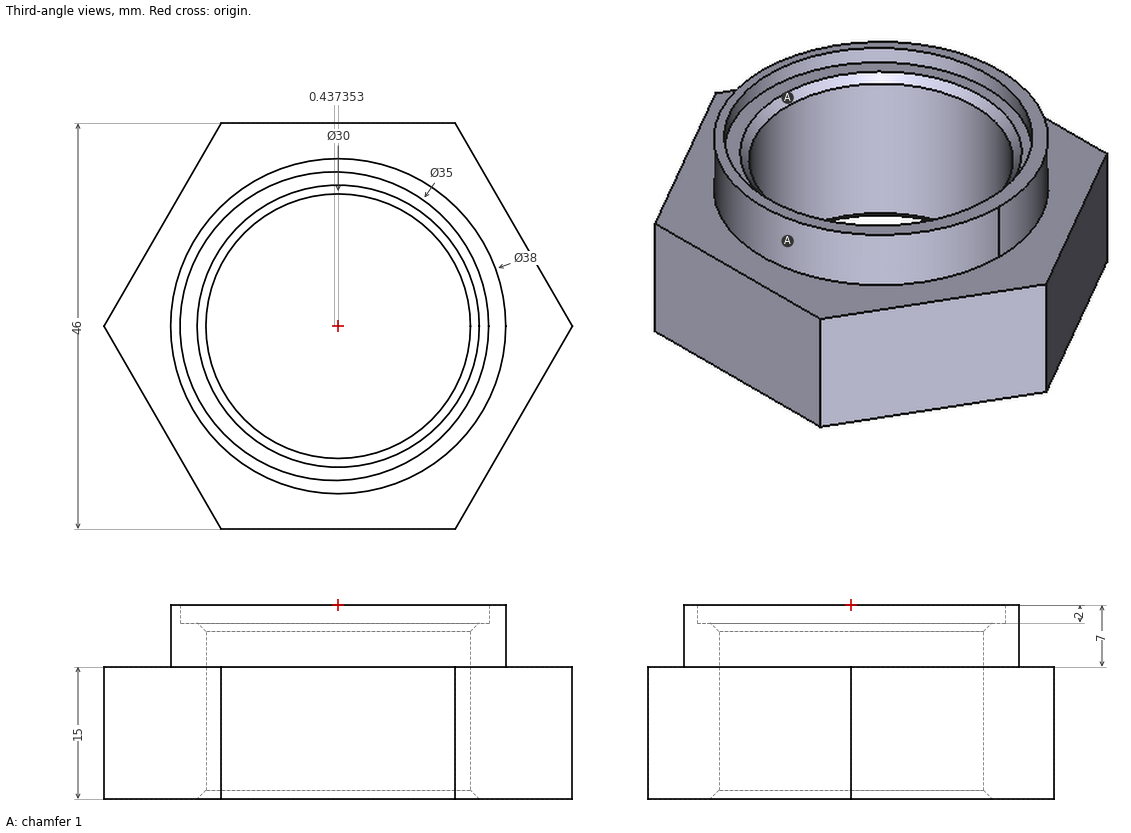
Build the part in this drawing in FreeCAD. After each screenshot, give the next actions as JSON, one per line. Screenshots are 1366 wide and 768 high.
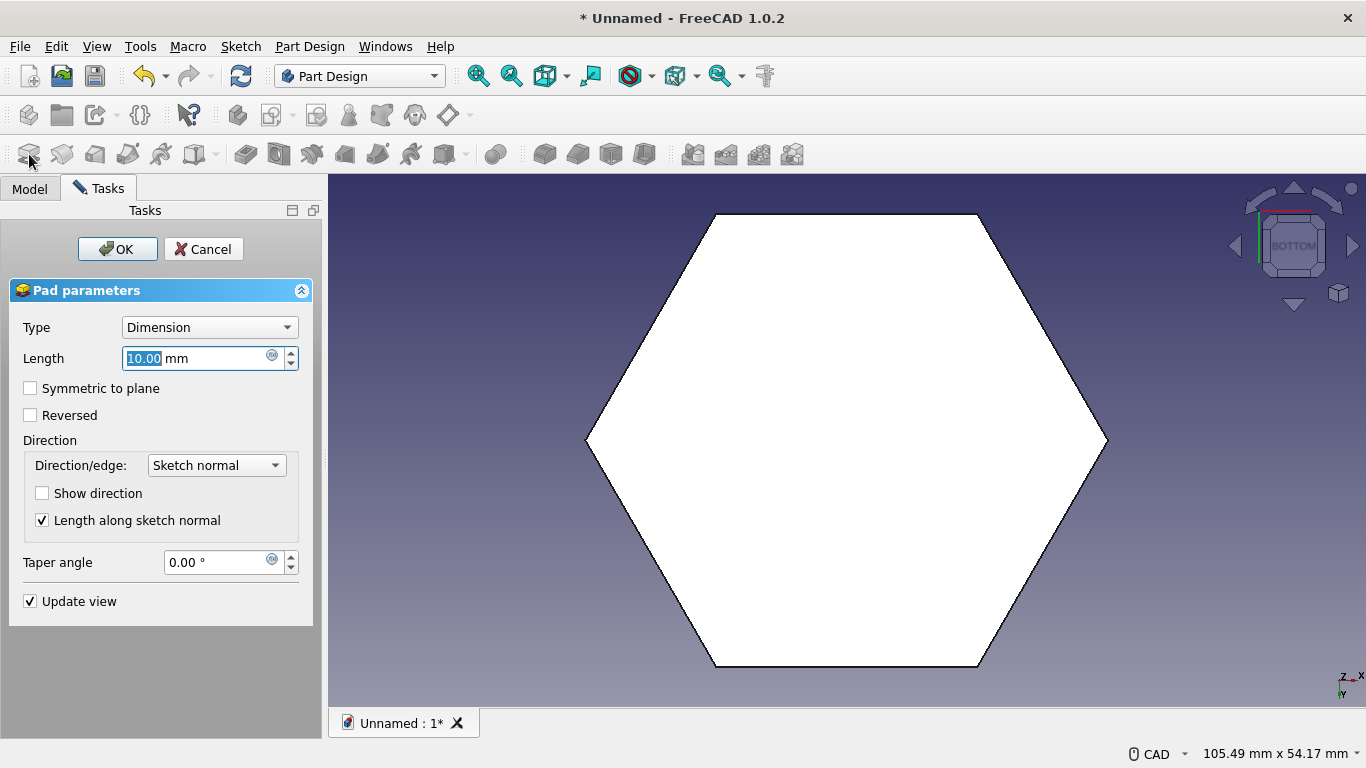
{"action": "type", "text": "15"}
{"action": "key", "text": "Tab"}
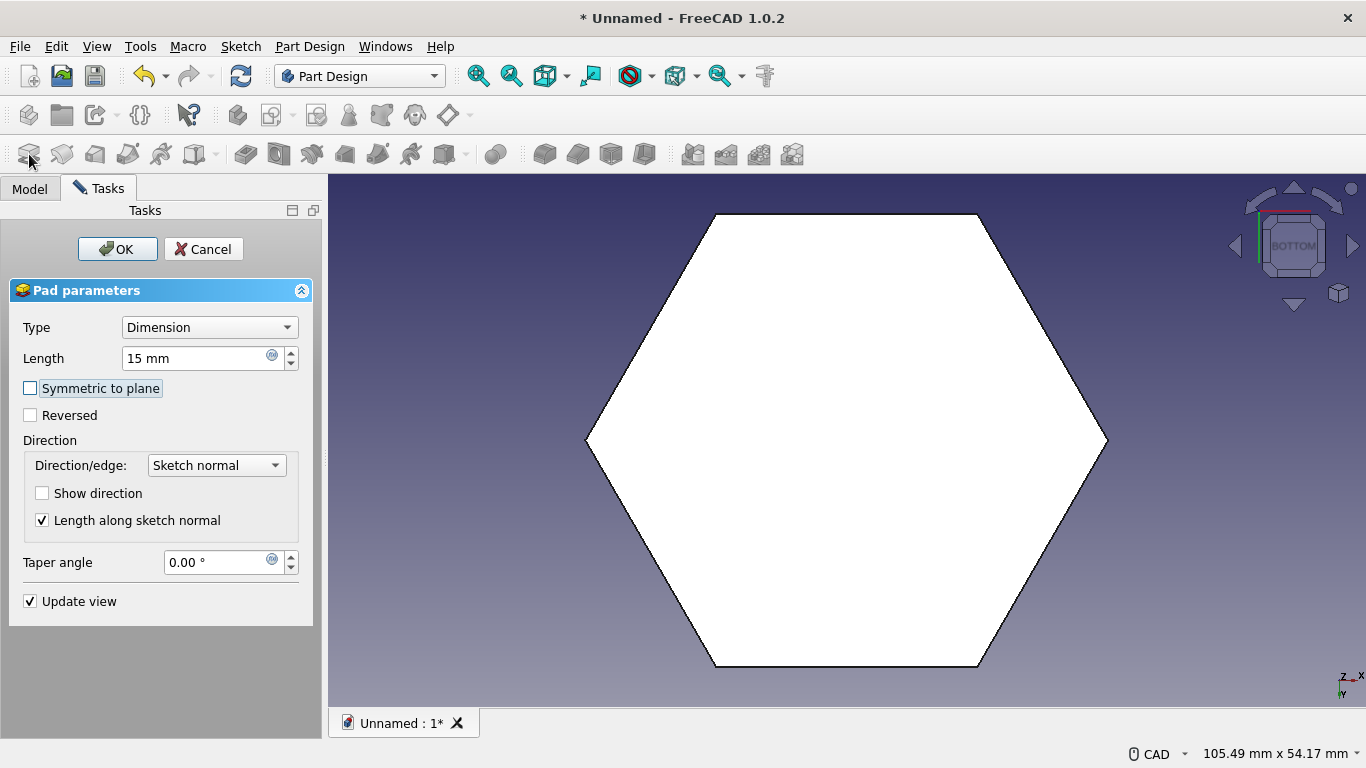
{"action": "left_click", "coordinate": [118, 249]}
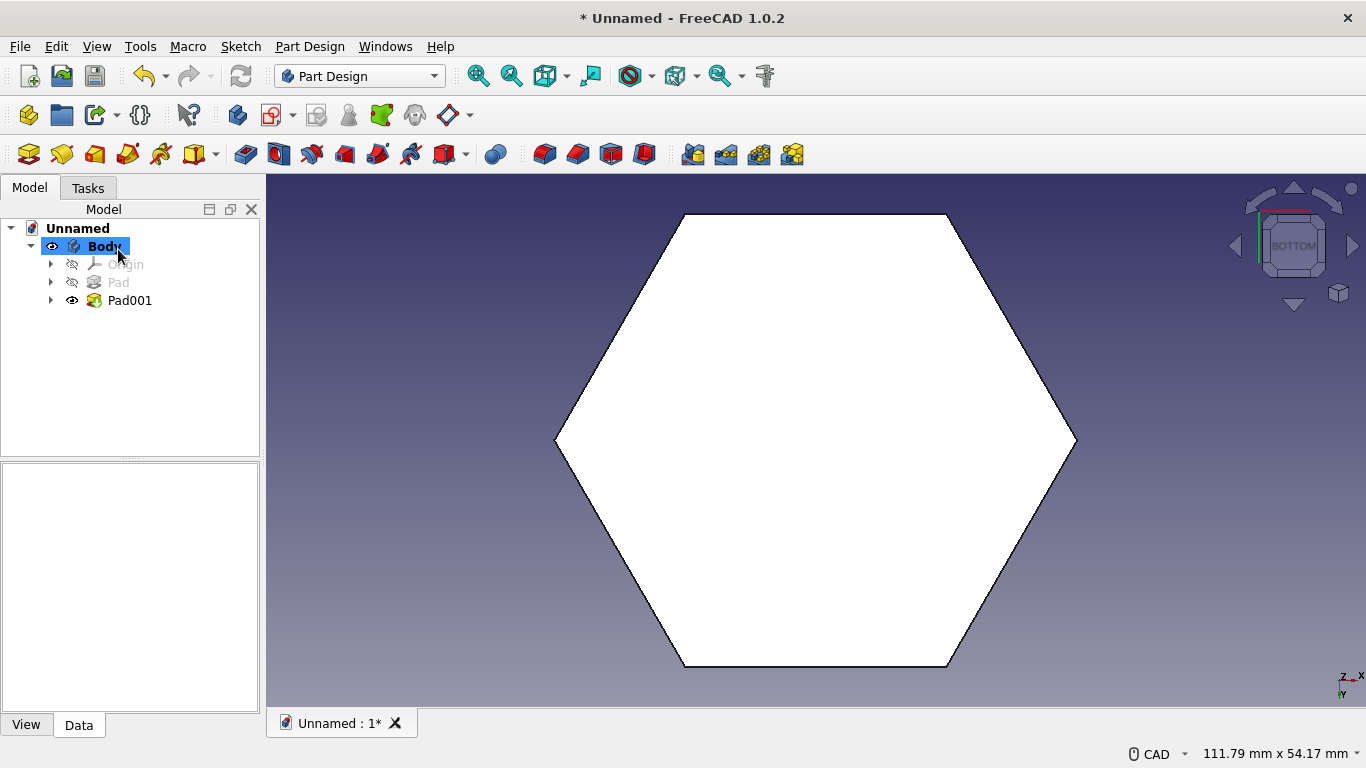
{"action": "left_click", "coordinate": [270, 116]}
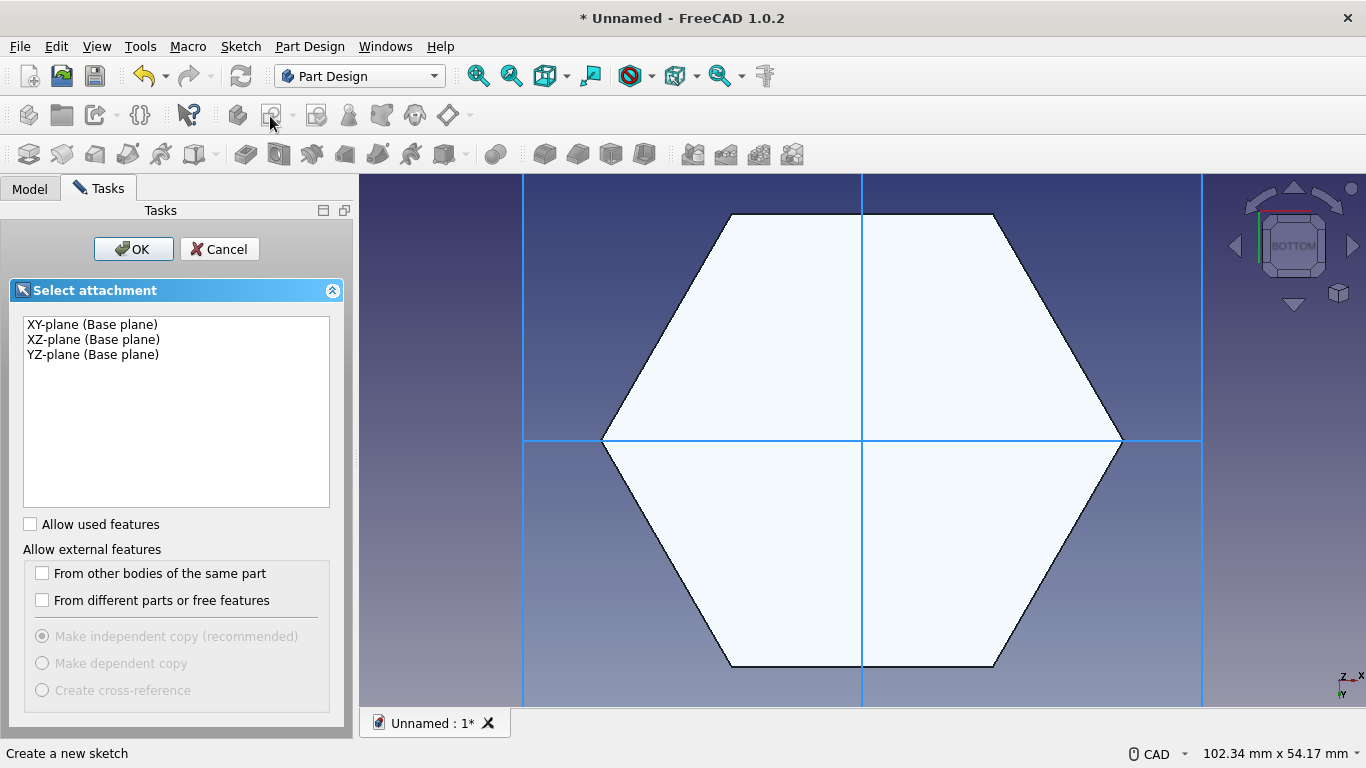
{"action": "left_click", "coordinate": [84, 324]}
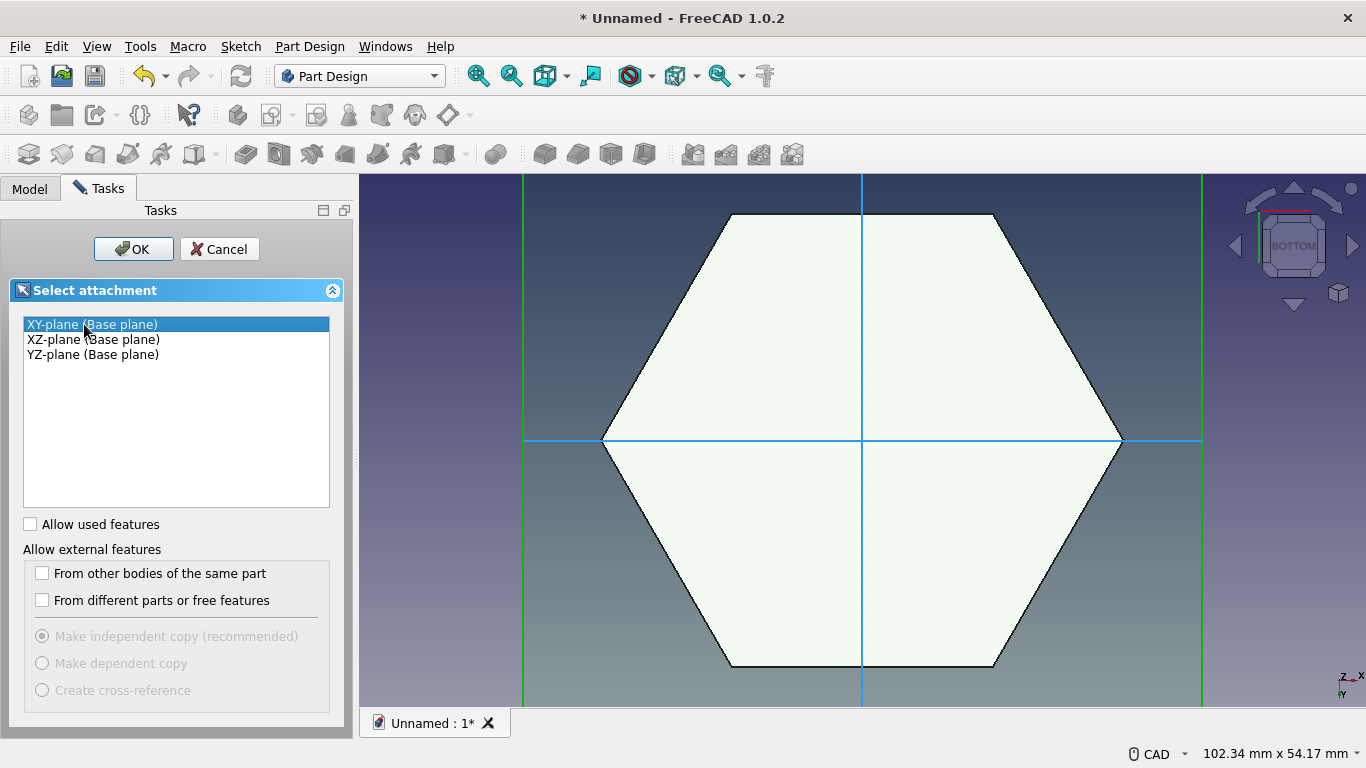
{"action": "left_click", "coordinate": [134, 249]}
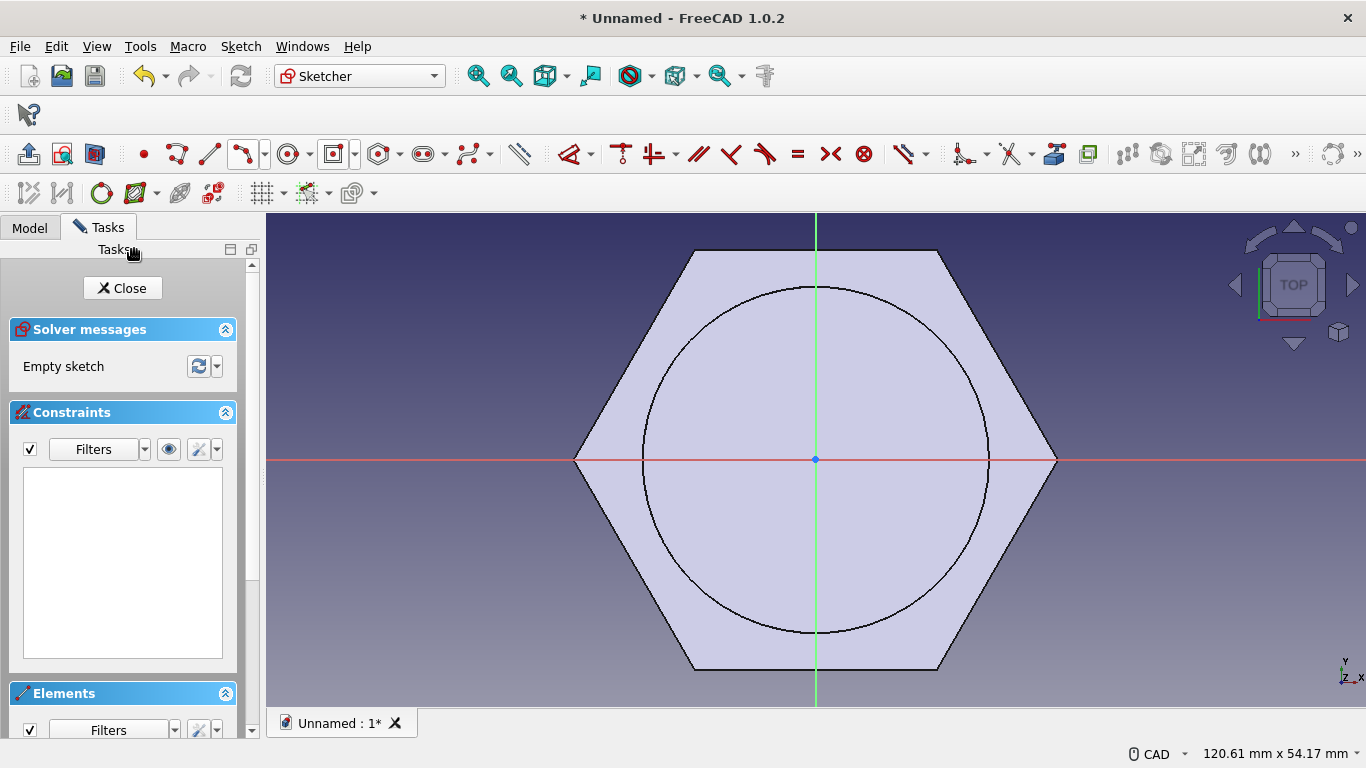
{"action": "left_click", "coordinate": [288, 154]}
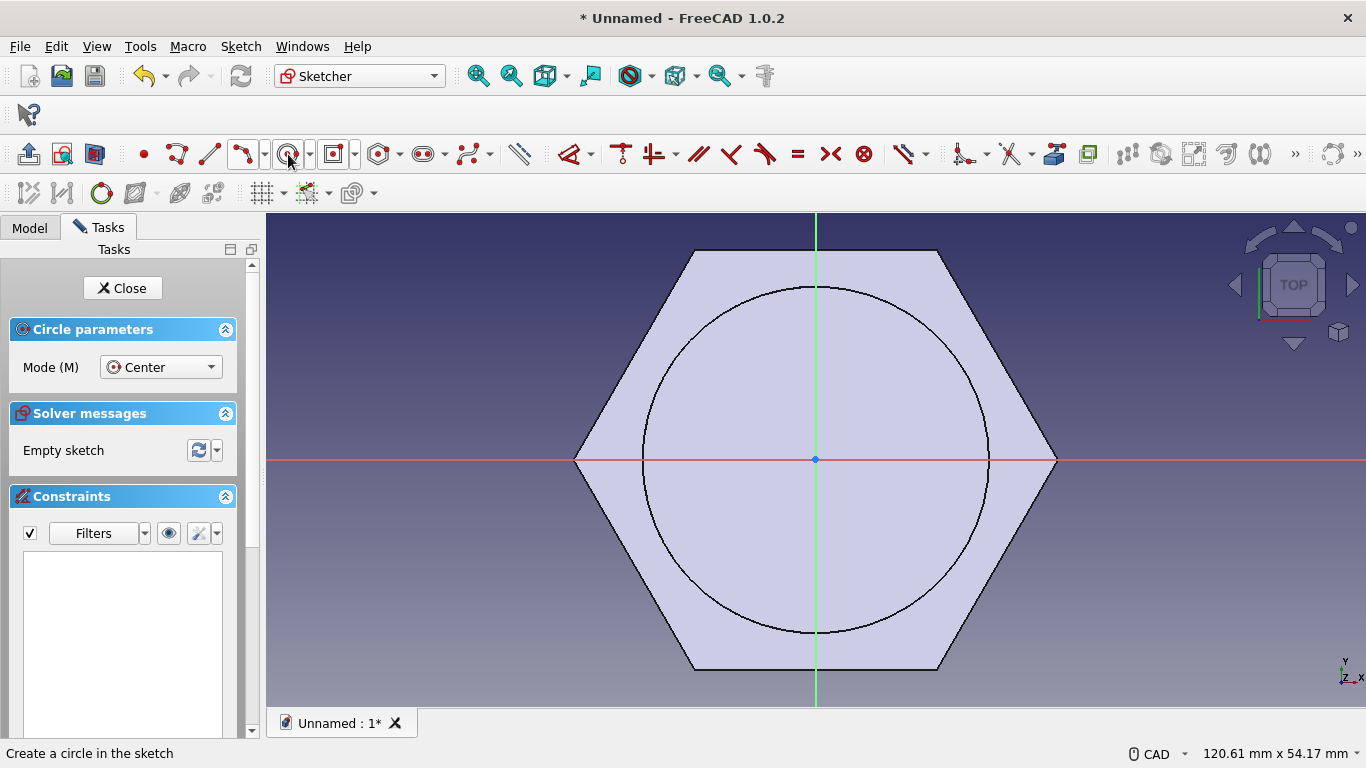
{"action": "scroll", "coordinate": [812, 460], "scroll_direction": "up", "scroll_amount": 7}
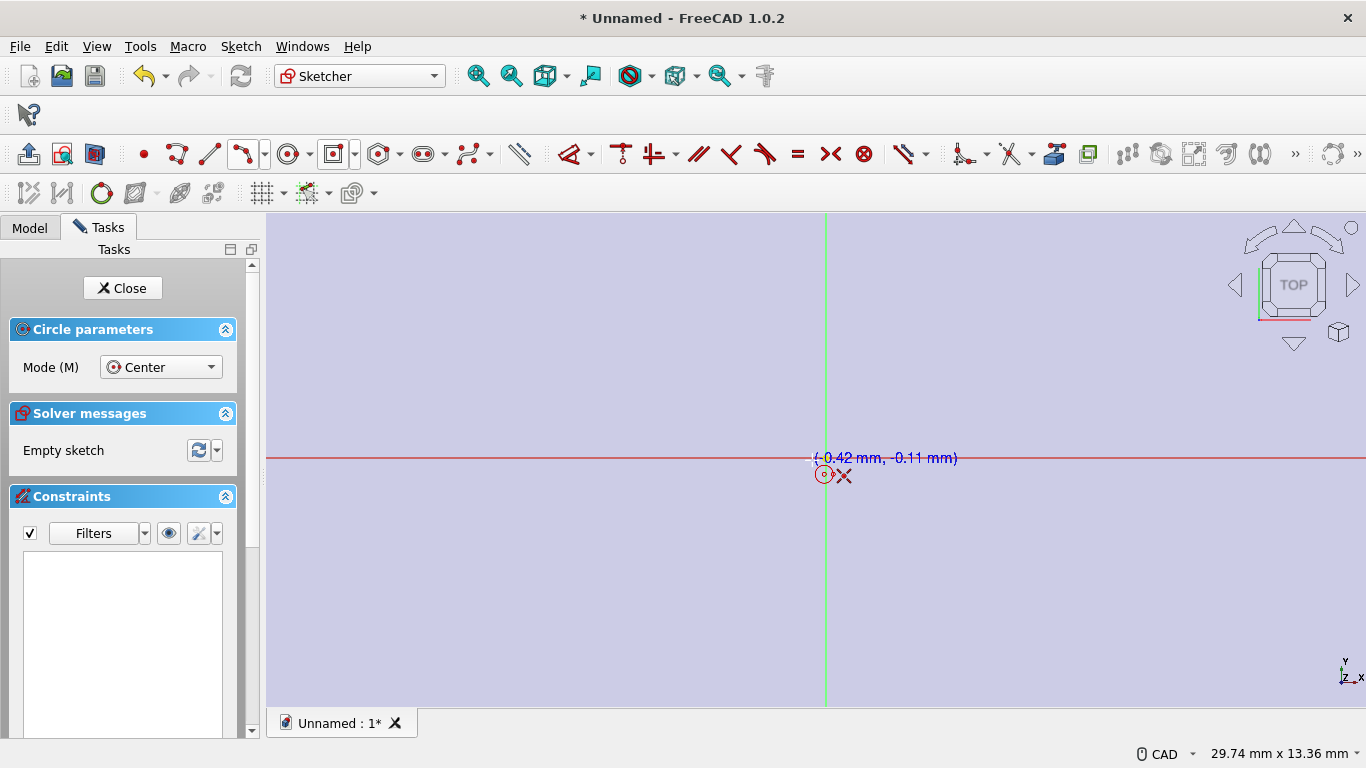
{"action": "left_click", "coordinate": [810, 458]}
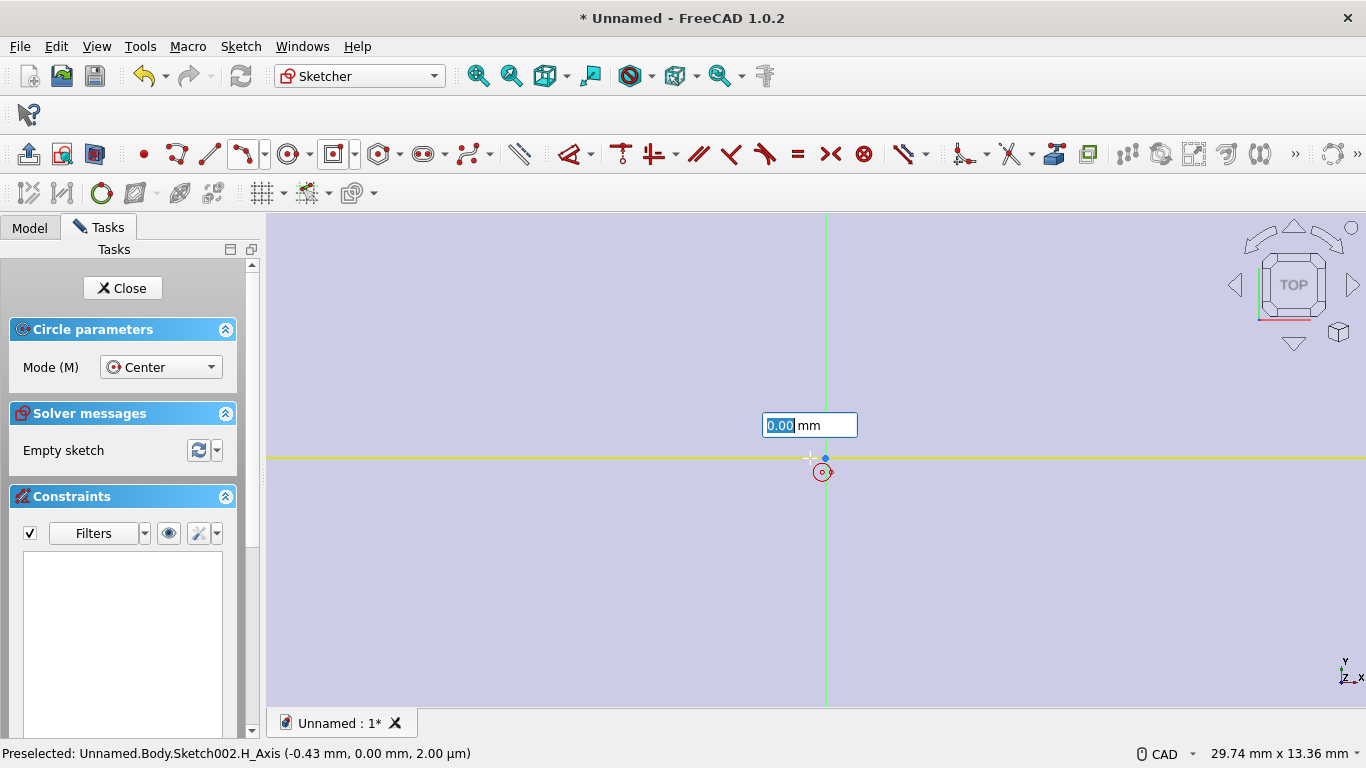
{"action": "scroll", "coordinate": [727, 461], "scroll_direction": "down", "scroll_amount": 7}
{"action": "mouse_move", "coordinate": [861, 348]}